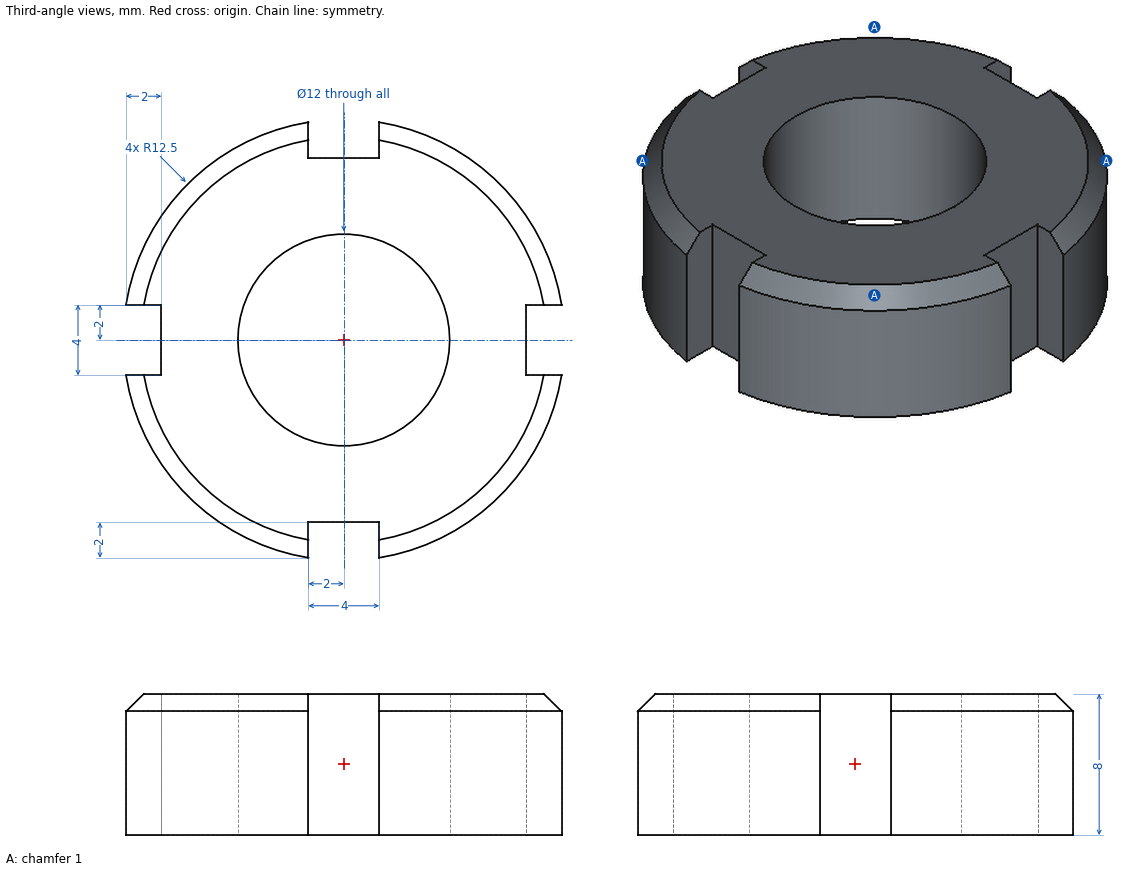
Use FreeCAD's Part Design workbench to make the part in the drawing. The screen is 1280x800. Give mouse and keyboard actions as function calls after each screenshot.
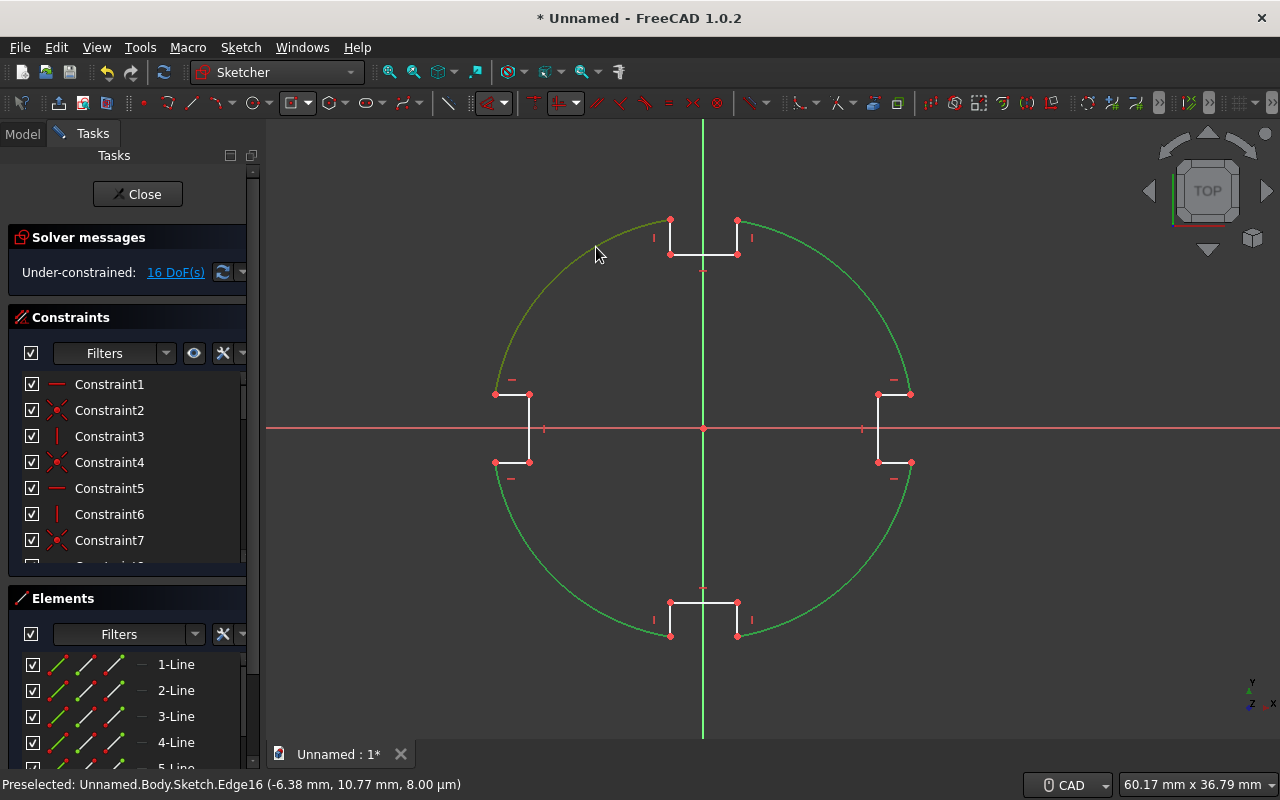
click(670, 104)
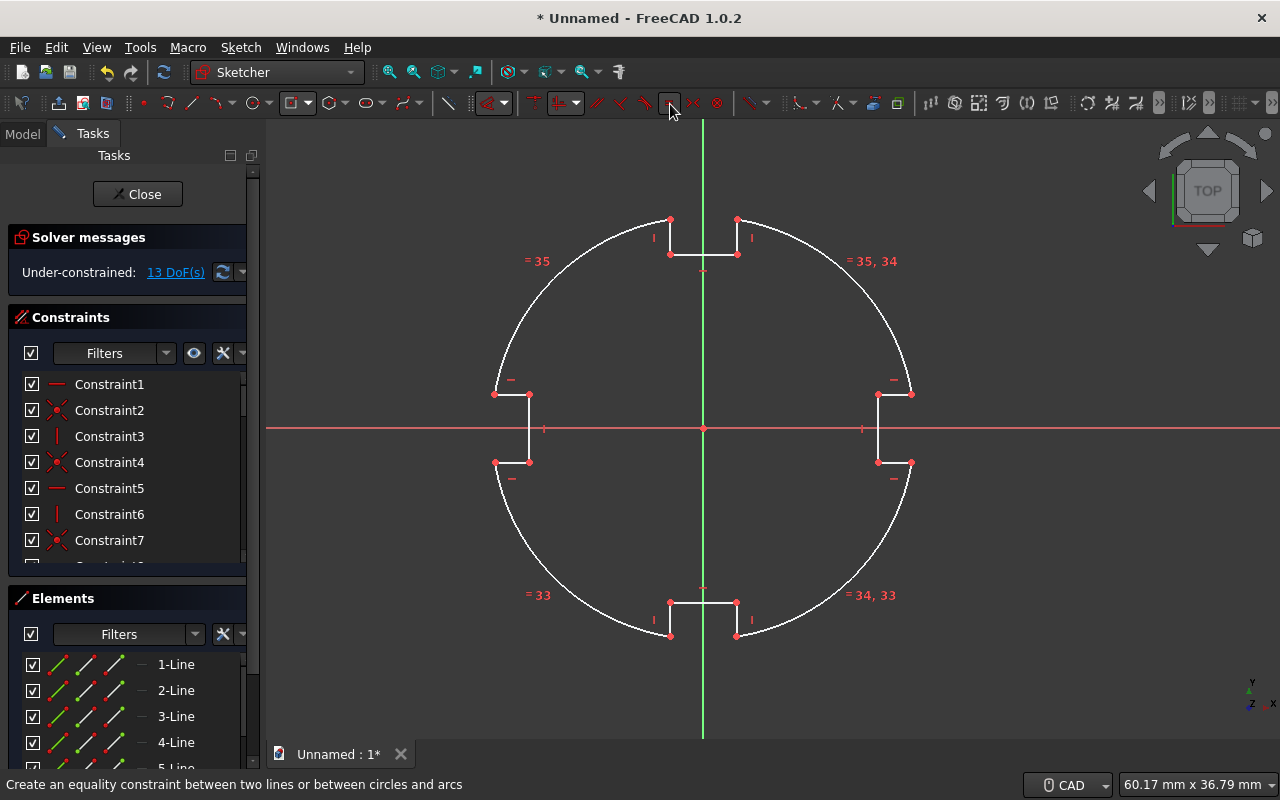
click(529, 463)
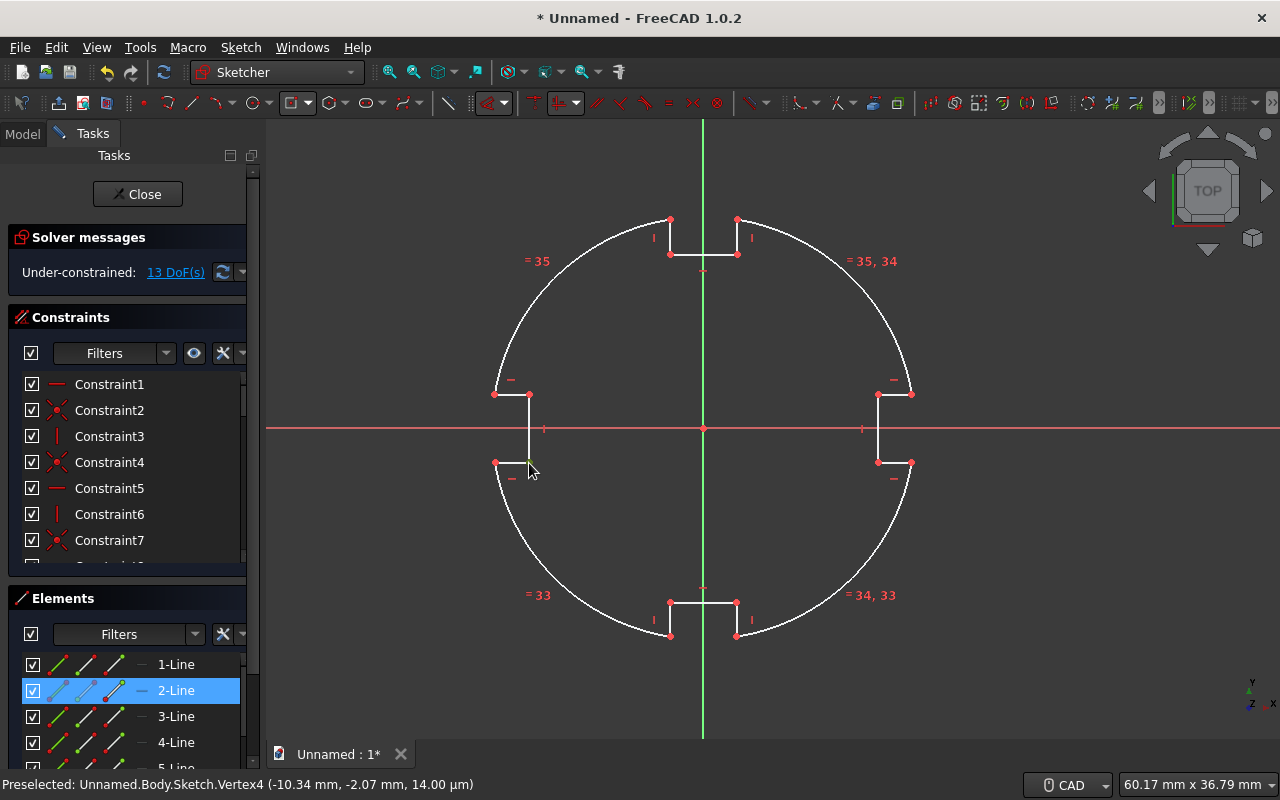
click(878, 463)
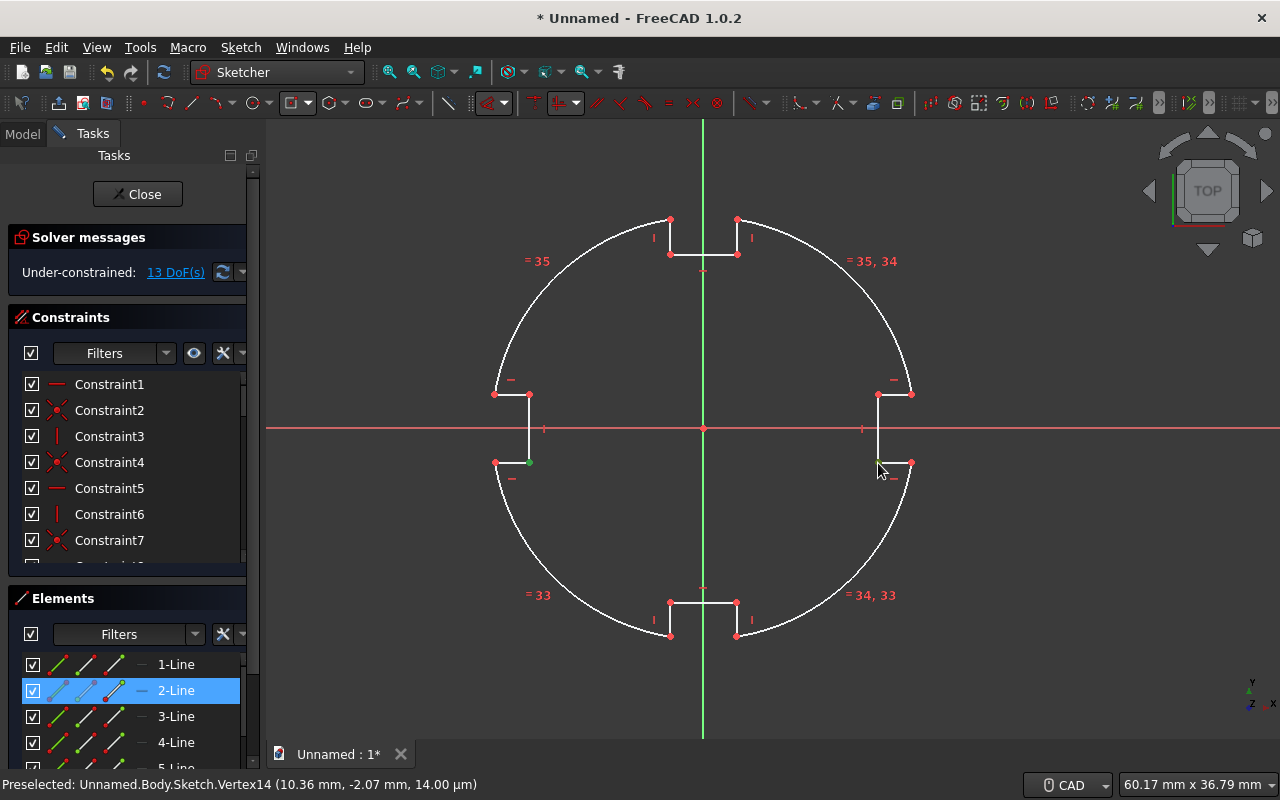
click(703, 671)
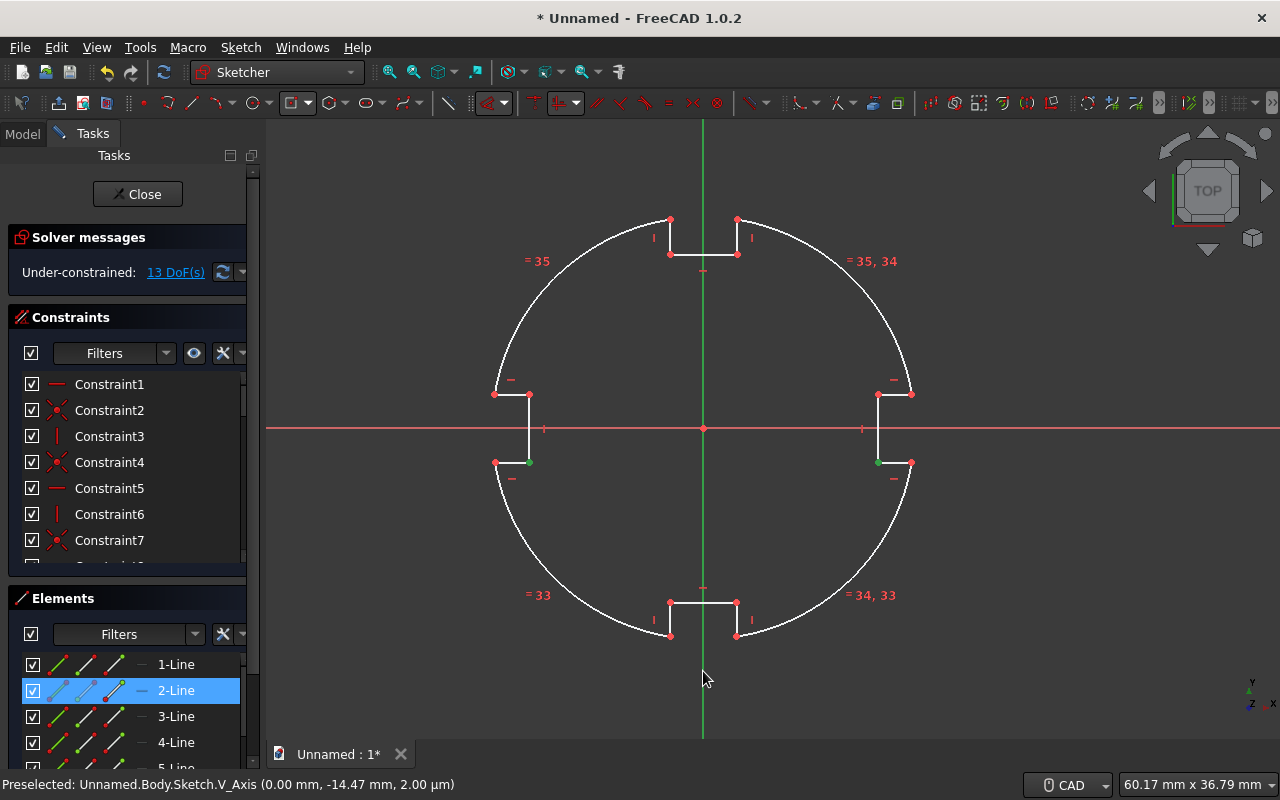
click(694, 104)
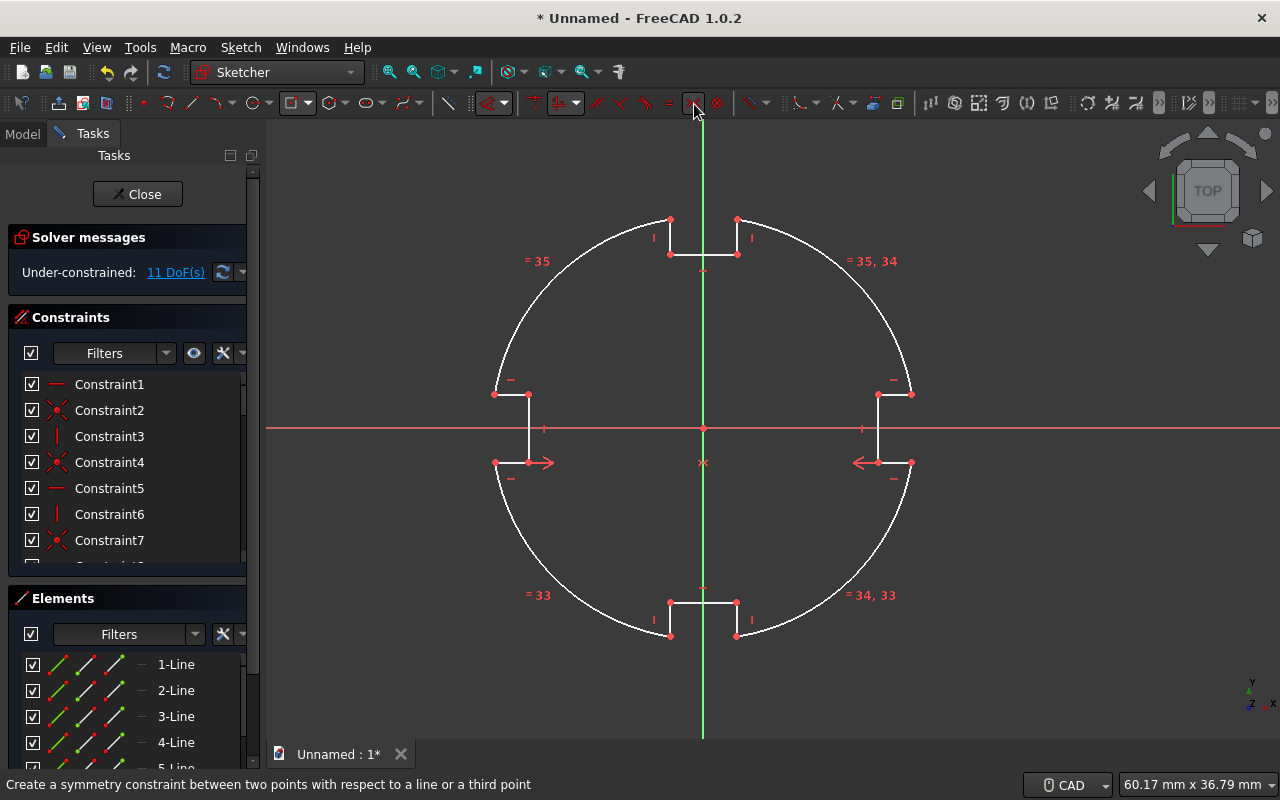
click(737, 603)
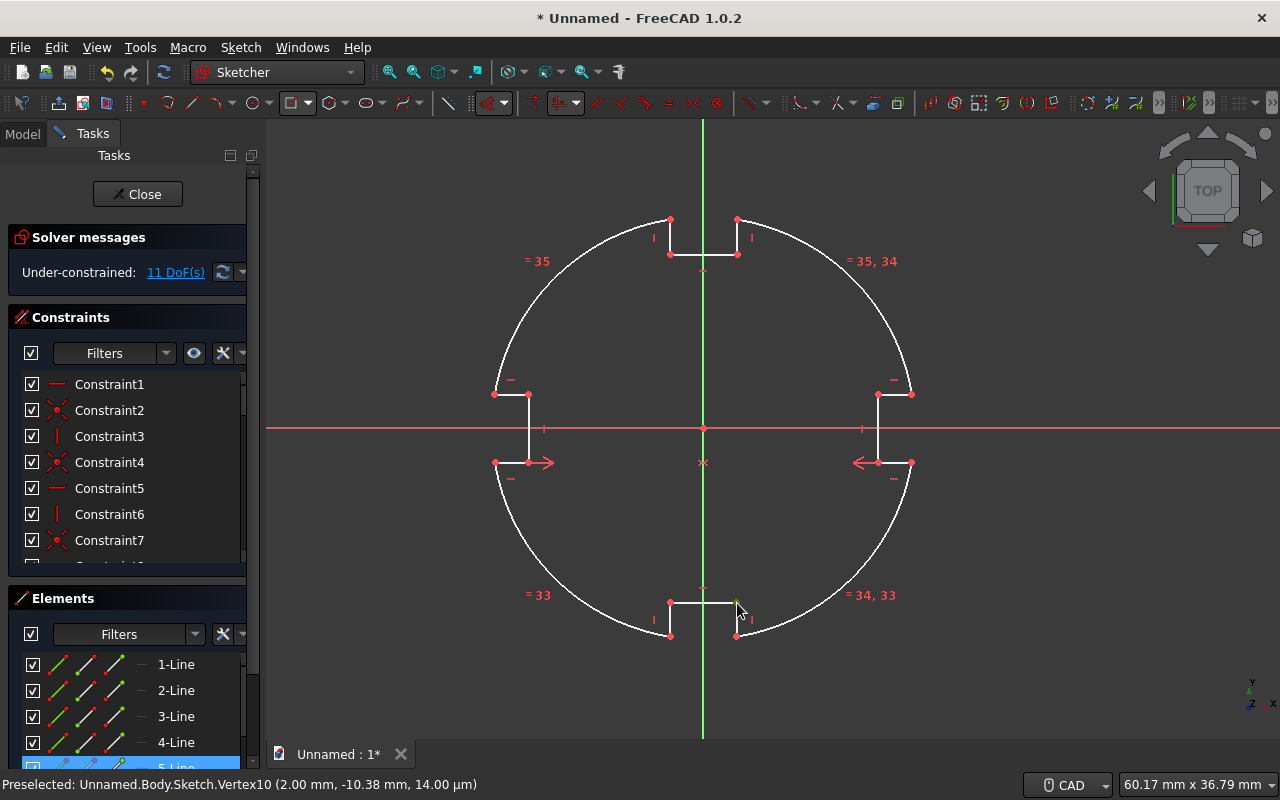
click(737, 255)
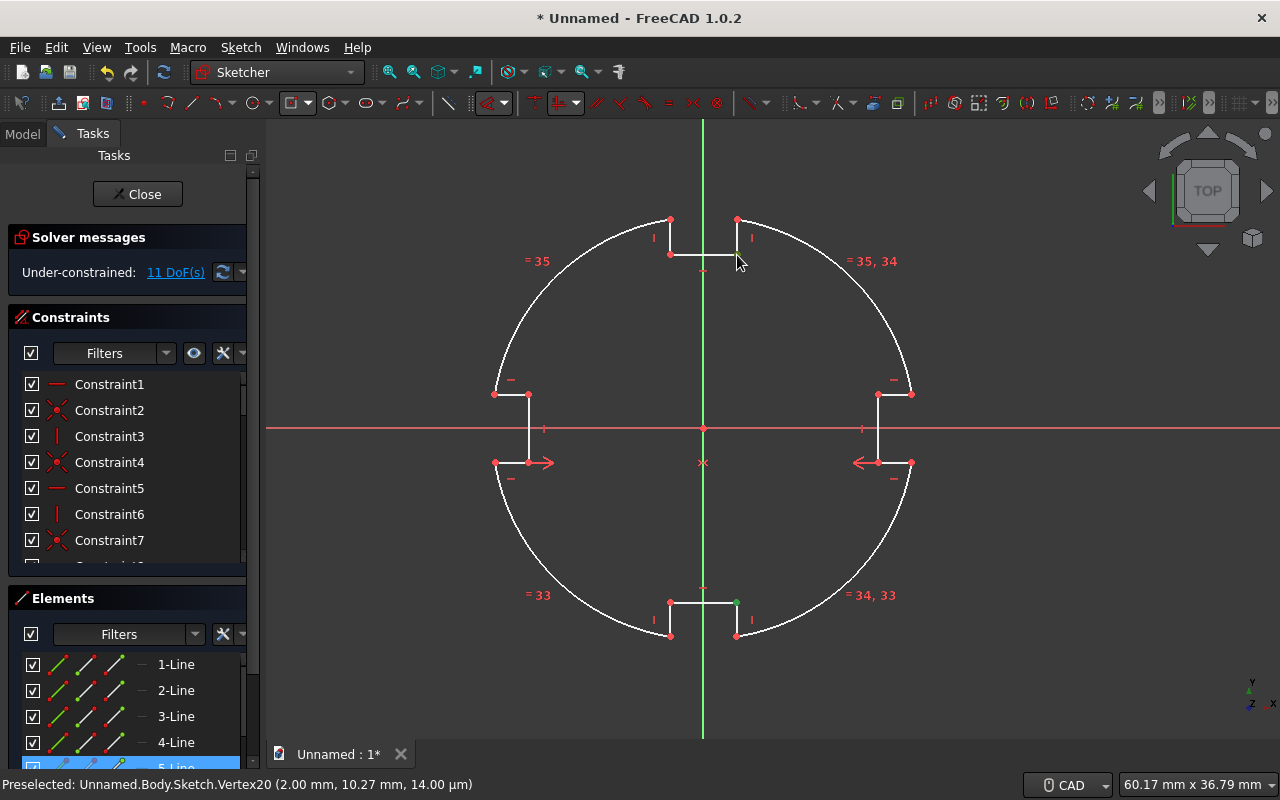
click(353, 428)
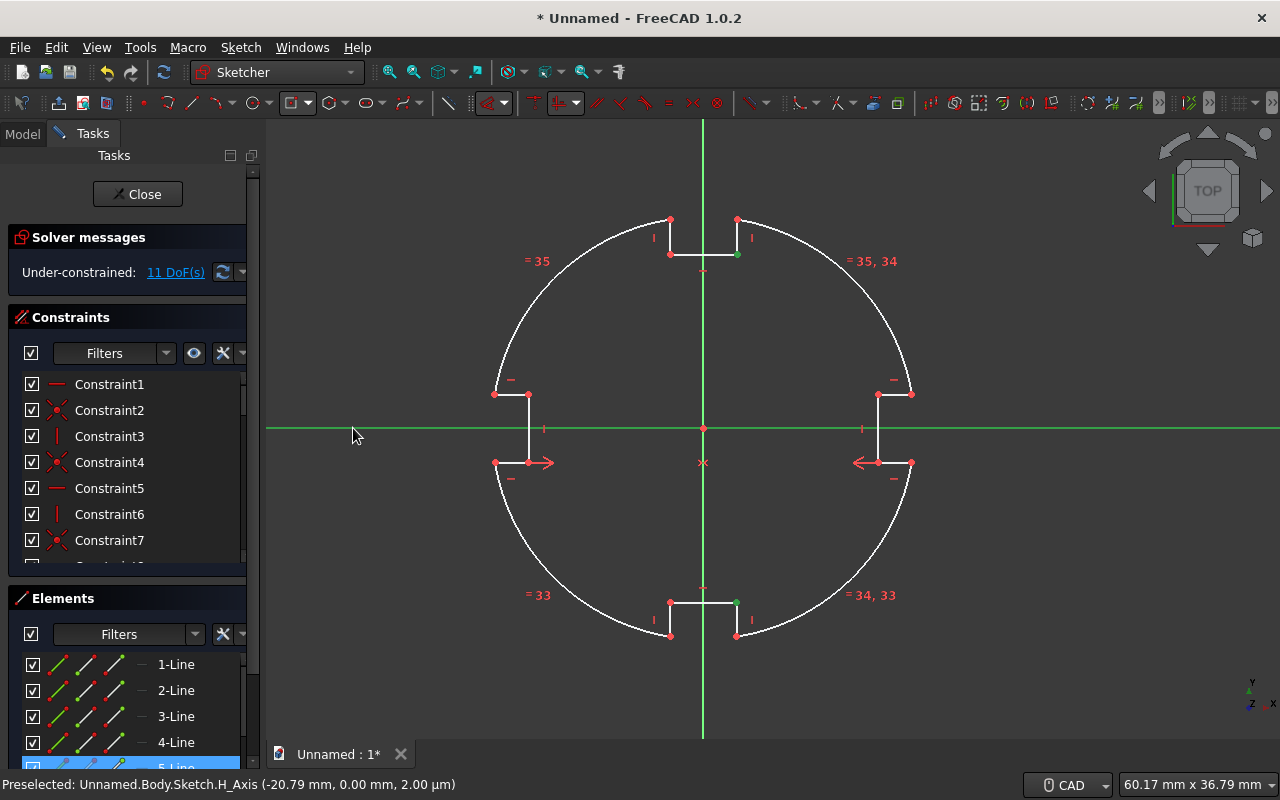
key(s)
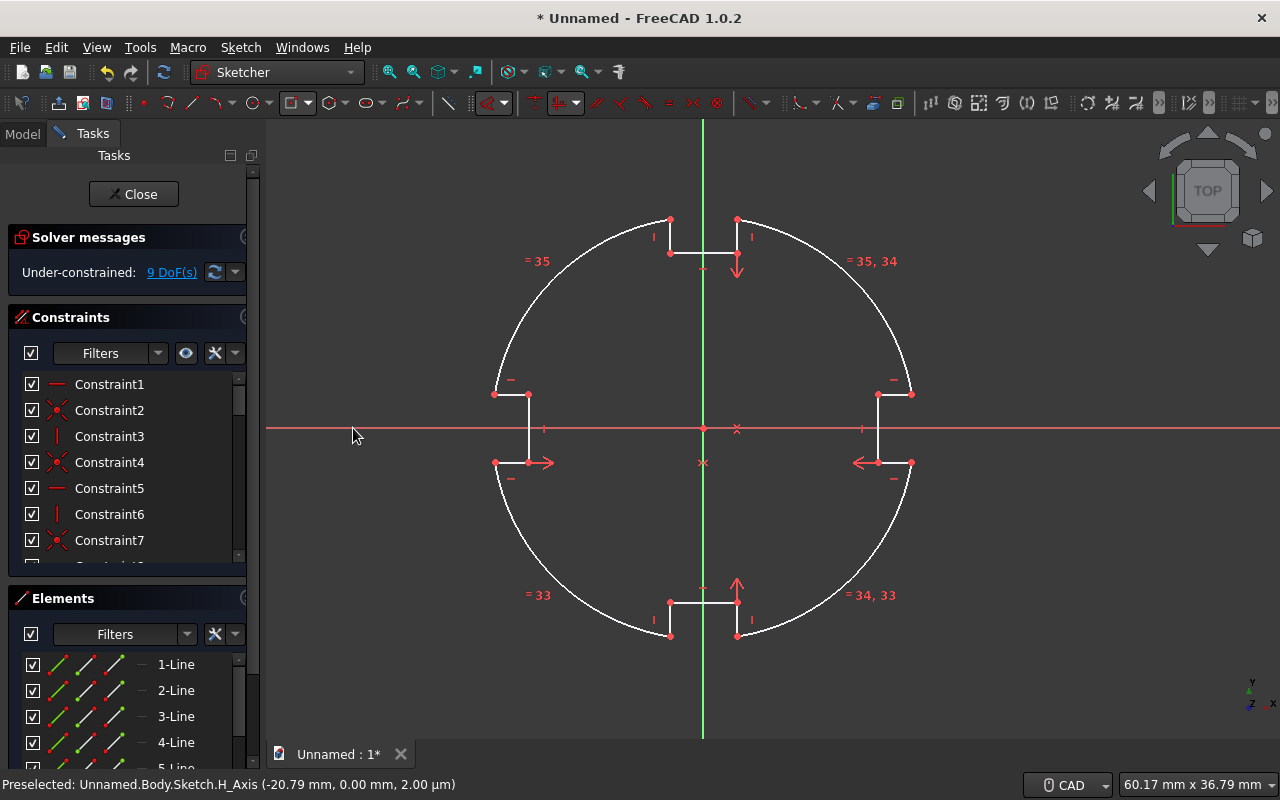
key(d)